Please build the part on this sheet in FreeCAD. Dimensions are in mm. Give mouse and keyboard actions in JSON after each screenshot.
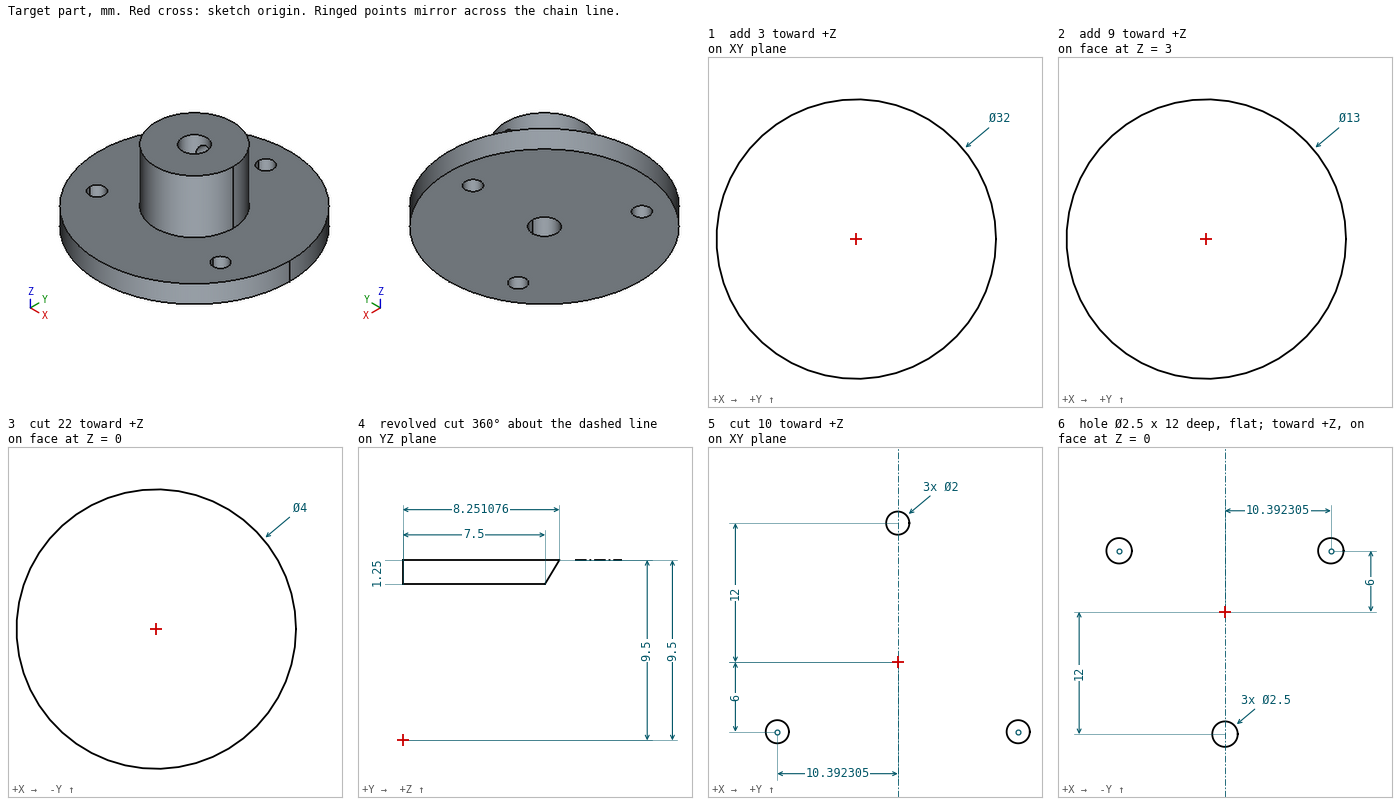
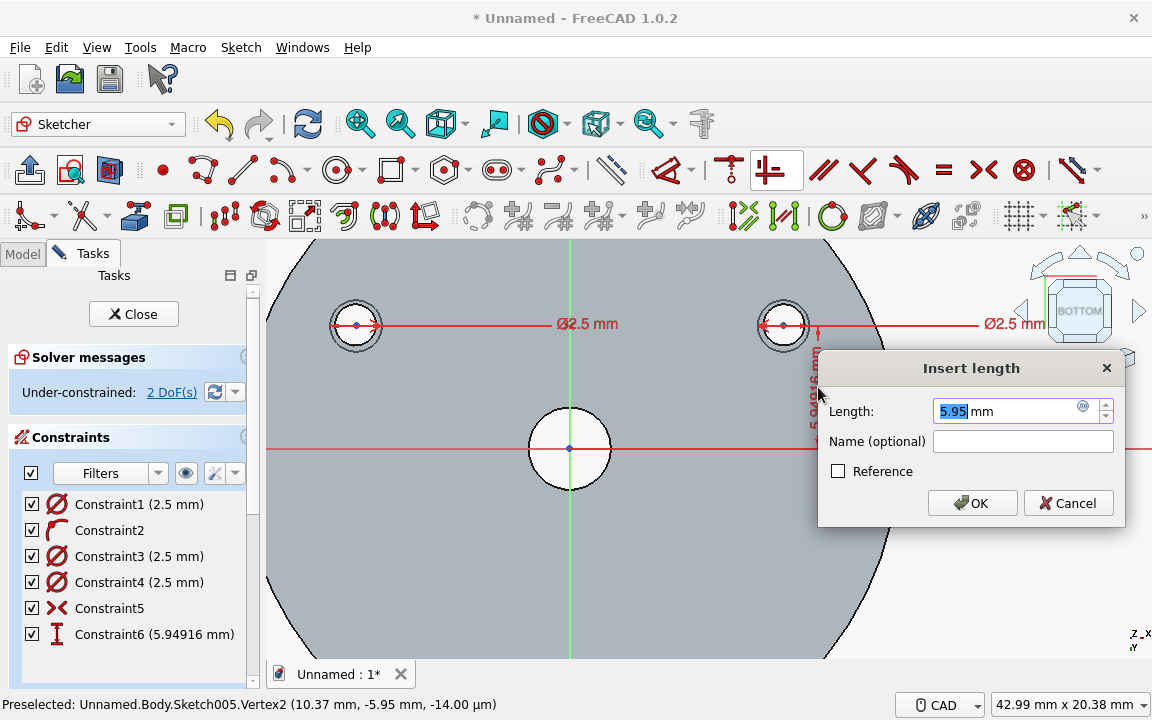
{"action": "type", "text": "6"}
{"action": "key", "text": "Return"}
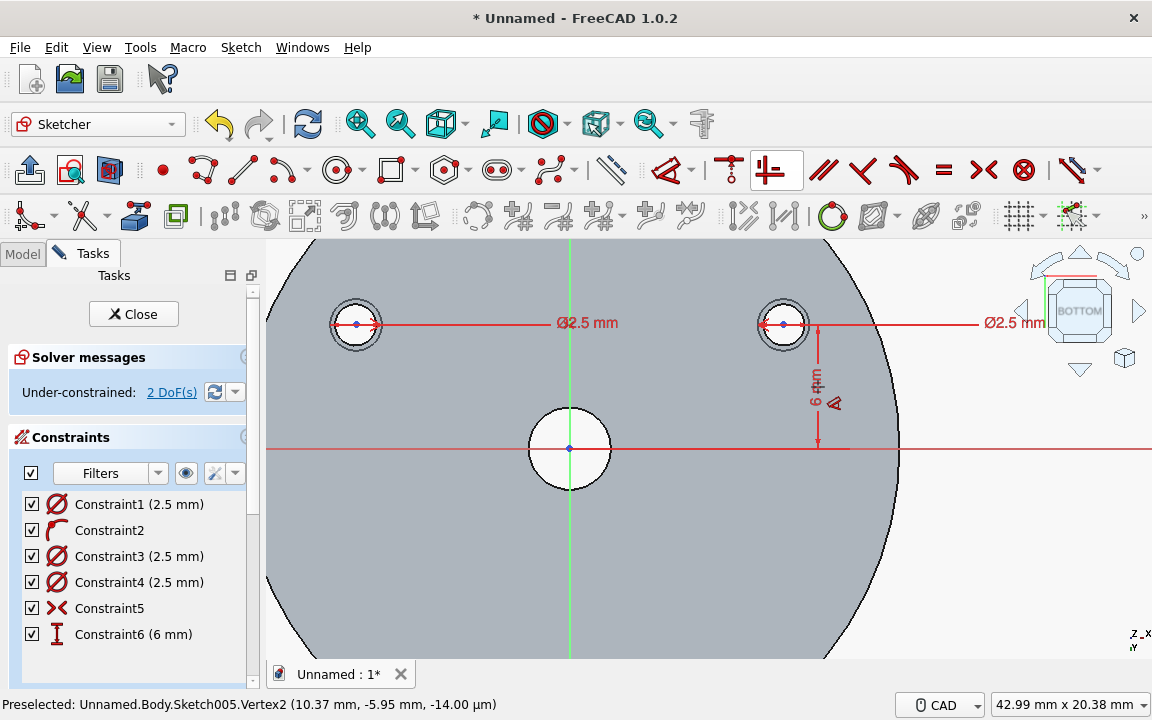
{"action": "scroll", "coordinate": [784, 324], "scroll_direction": "down", "scroll_amount": 2}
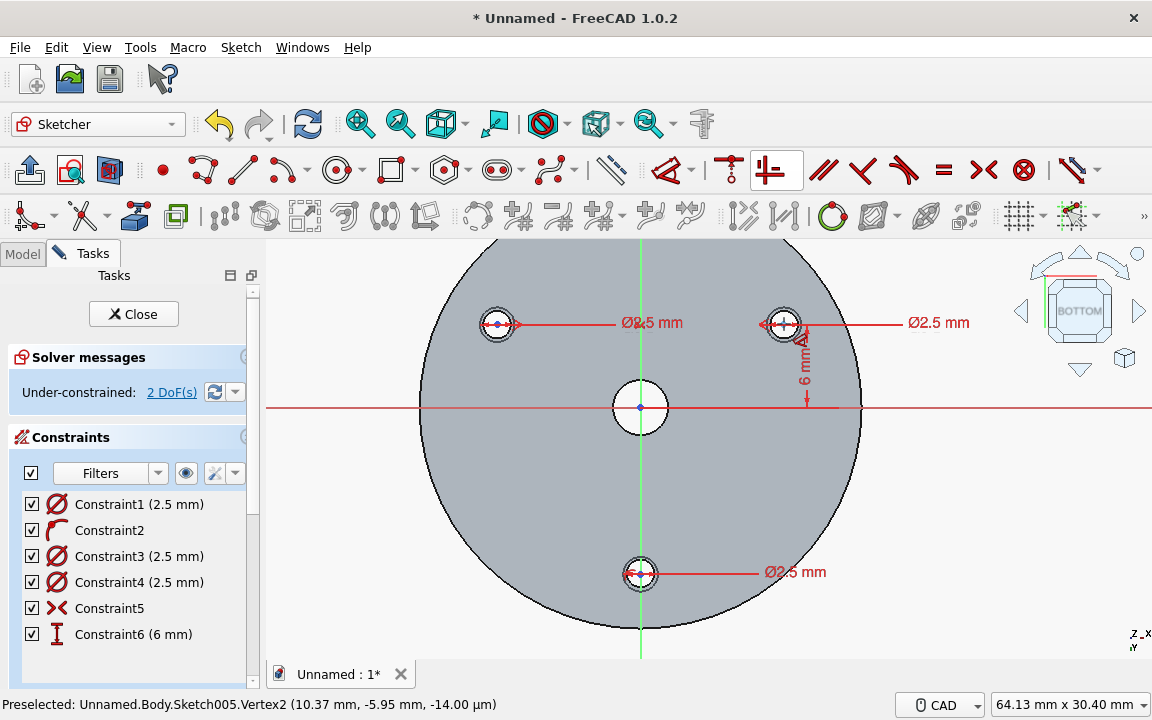
{"action": "left_click", "coordinate": [641, 574]}
{"action": "left_click", "coordinate": [675, 491]}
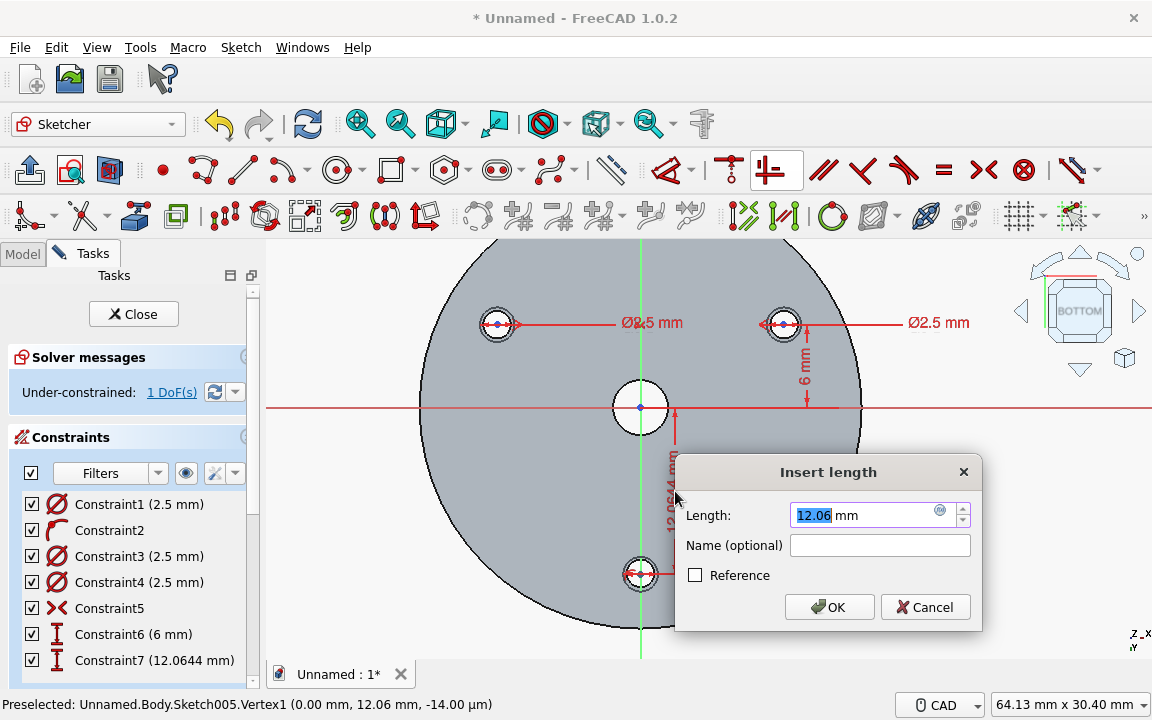
{"action": "type", "text": "12"}
{"action": "key", "text": "Return"}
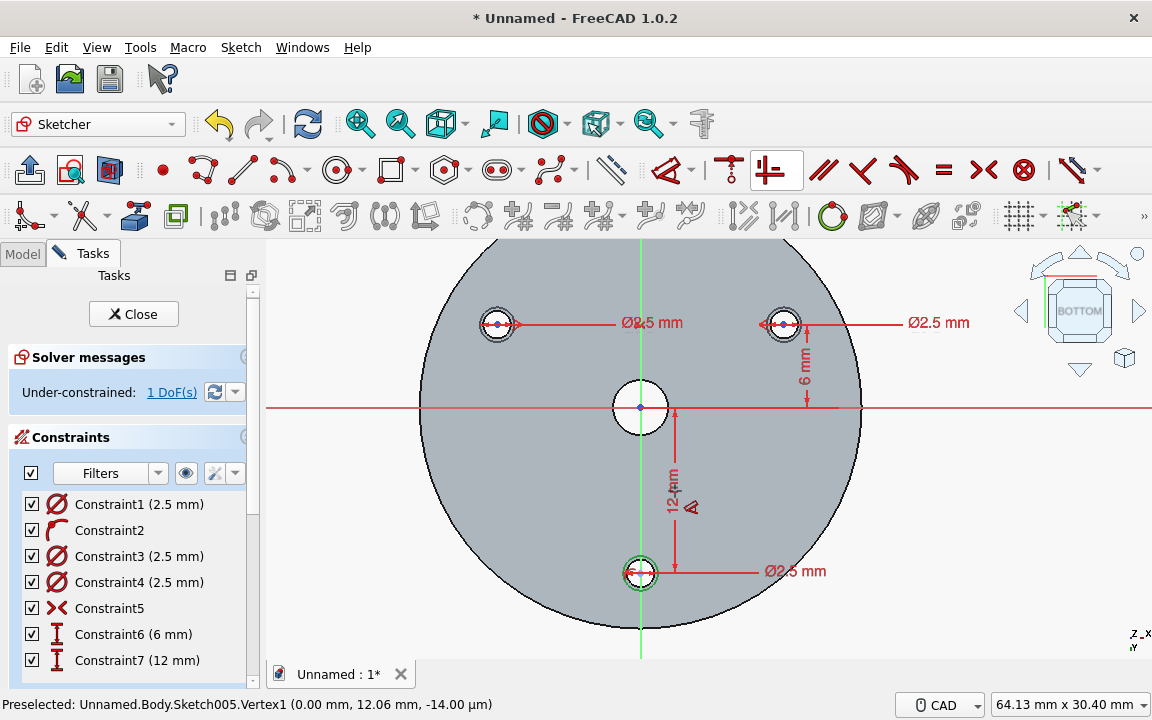
{"action": "left_click", "coordinate": [784, 325]}
{"action": "left_click", "coordinate": [712, 291]}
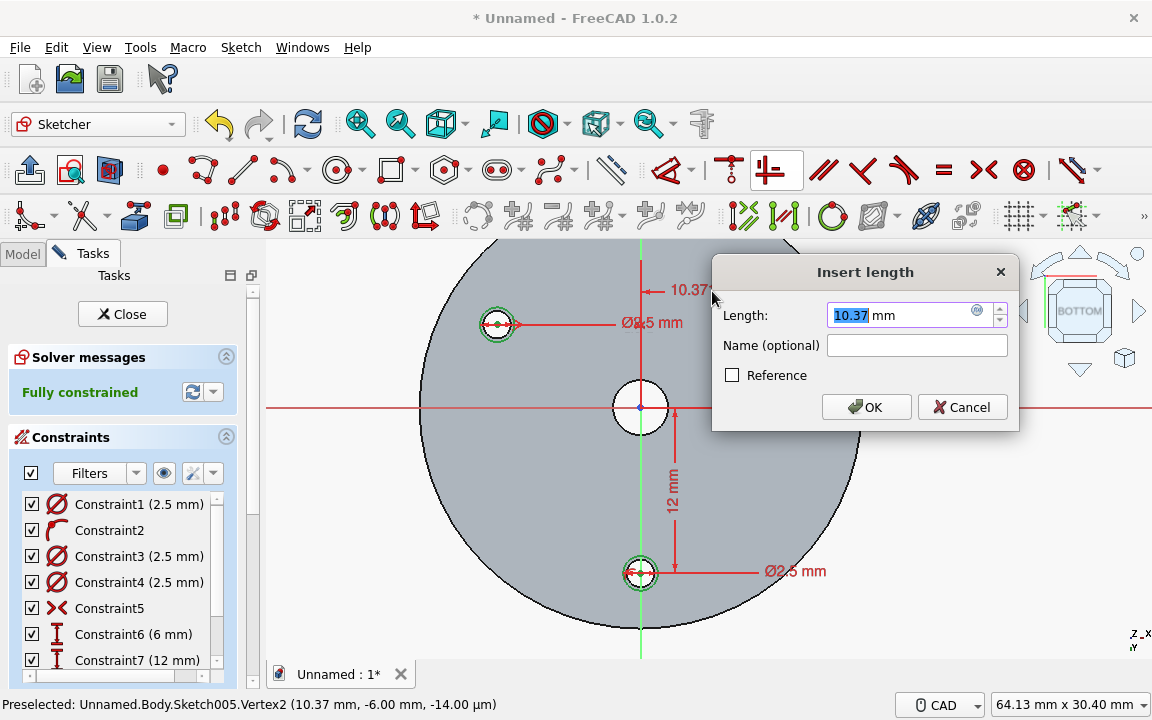
{"action": "type", "text": "10.392305"}
{"action": "key", "text": "Return"}
{"action": "key", "text": "Escape"}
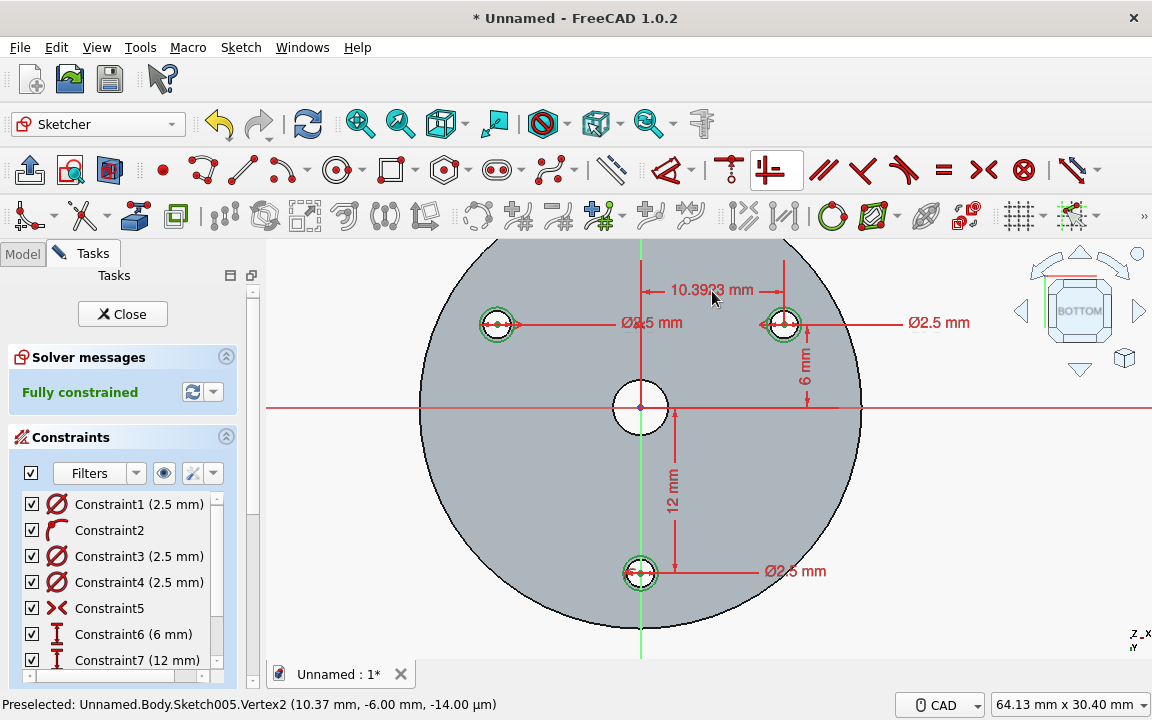
{"action": "left_click", "coordinate": [123, 314]}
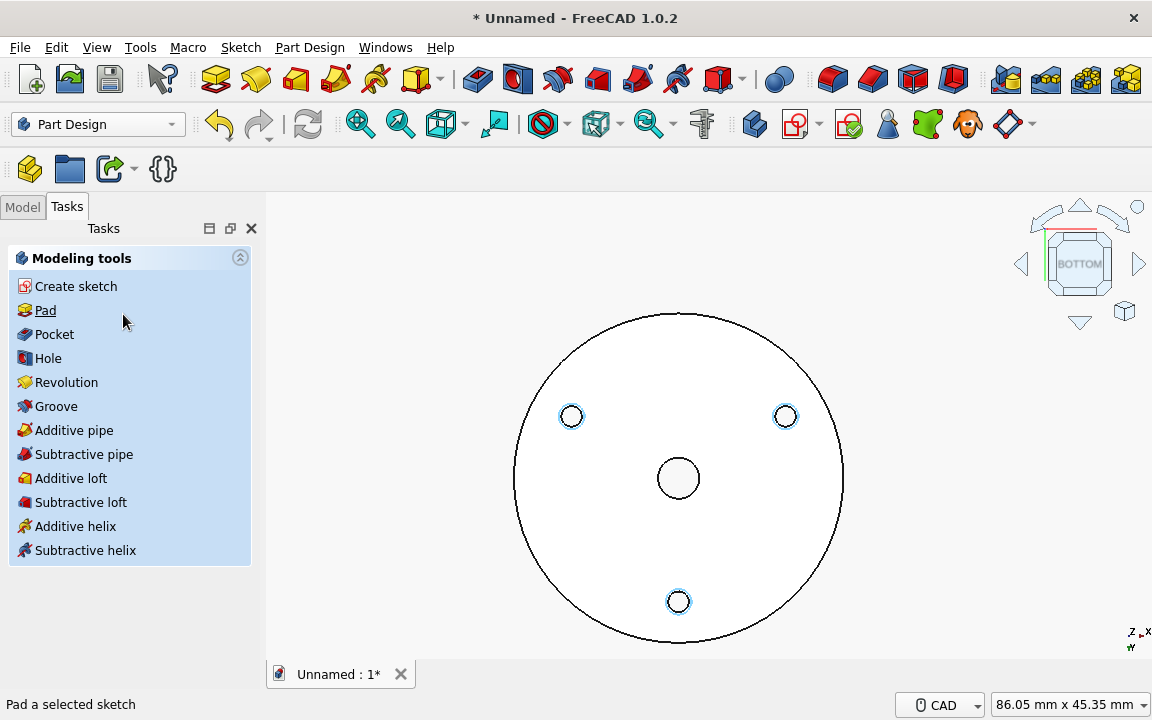
{"action": "left_click", "coordinate": [518, 80]}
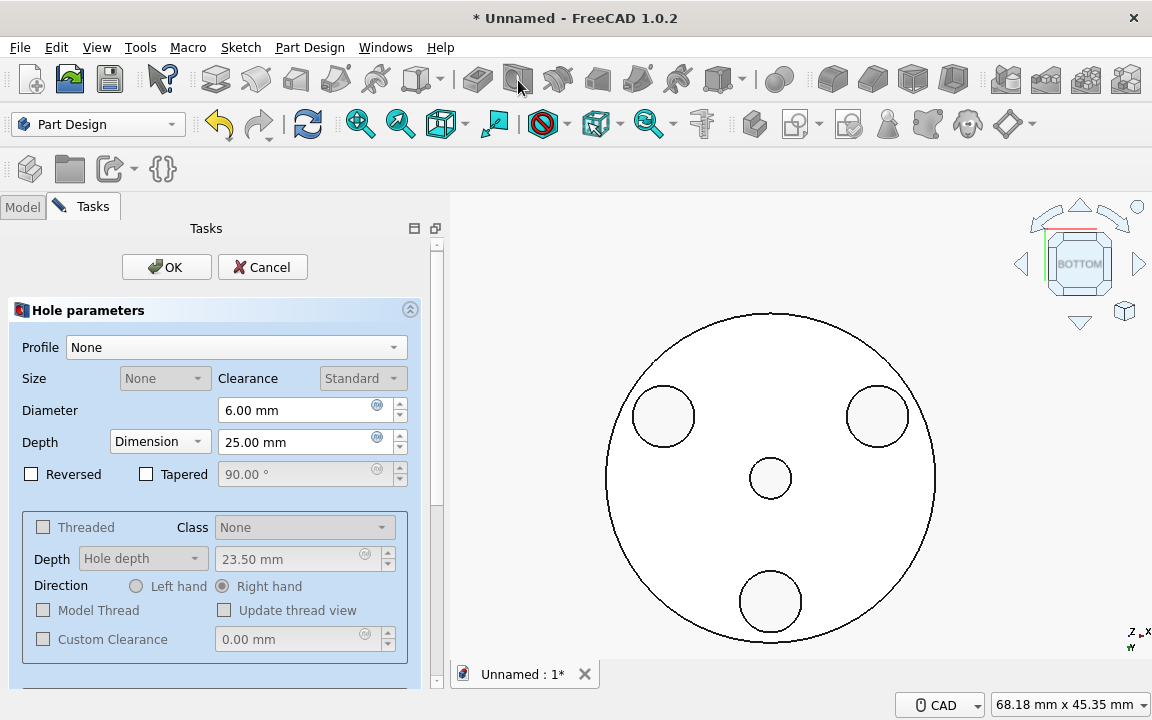
{"action": "triple_click", "coordinate": [305, 410]}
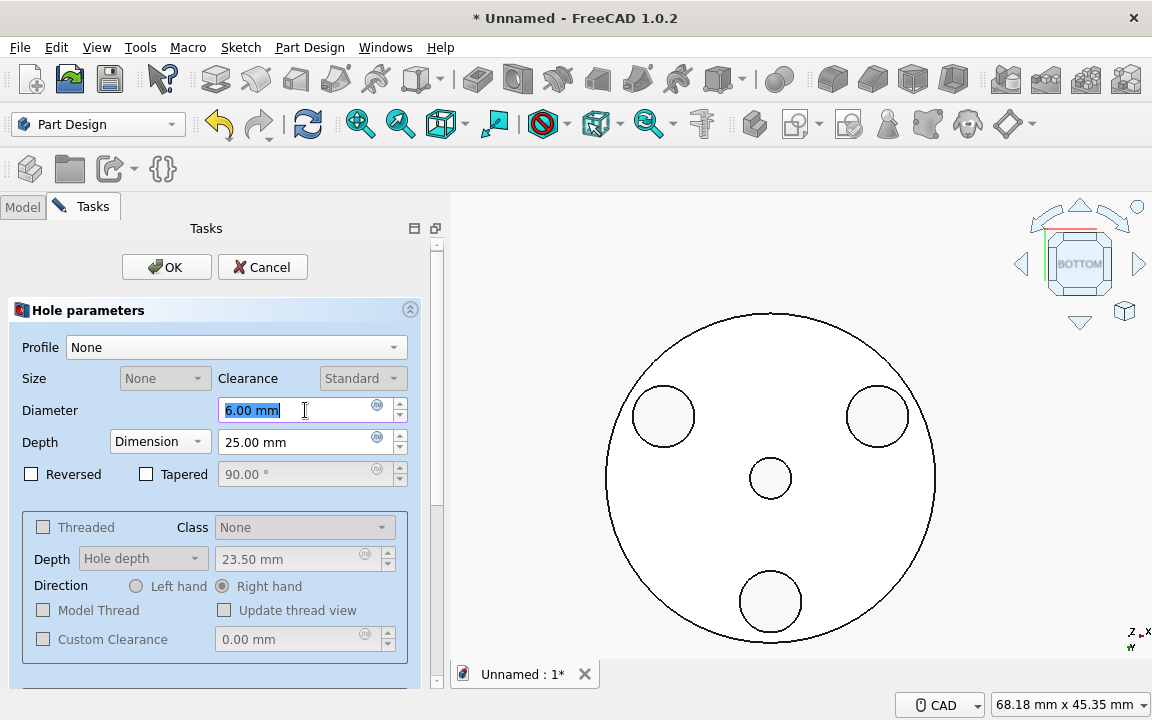
{"action": "type", "text": "2.5"}
{"action": "key", "text": "Tab"}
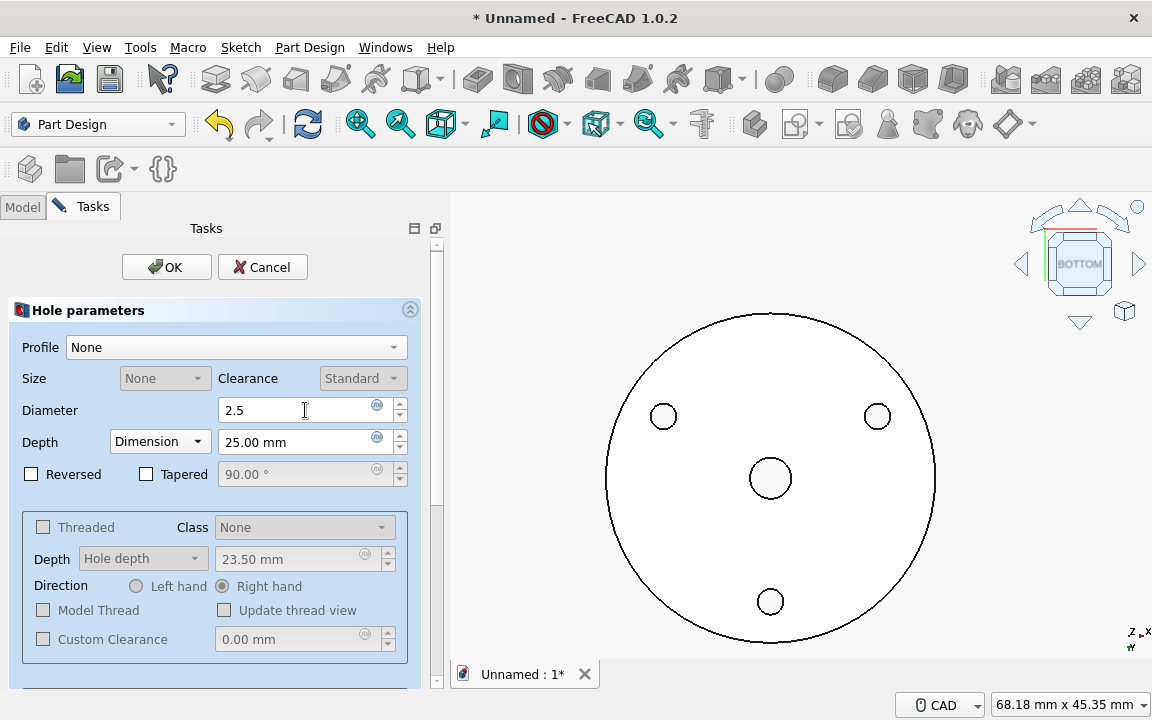
{"action": "triple_click", "coordinate": [305, 442]}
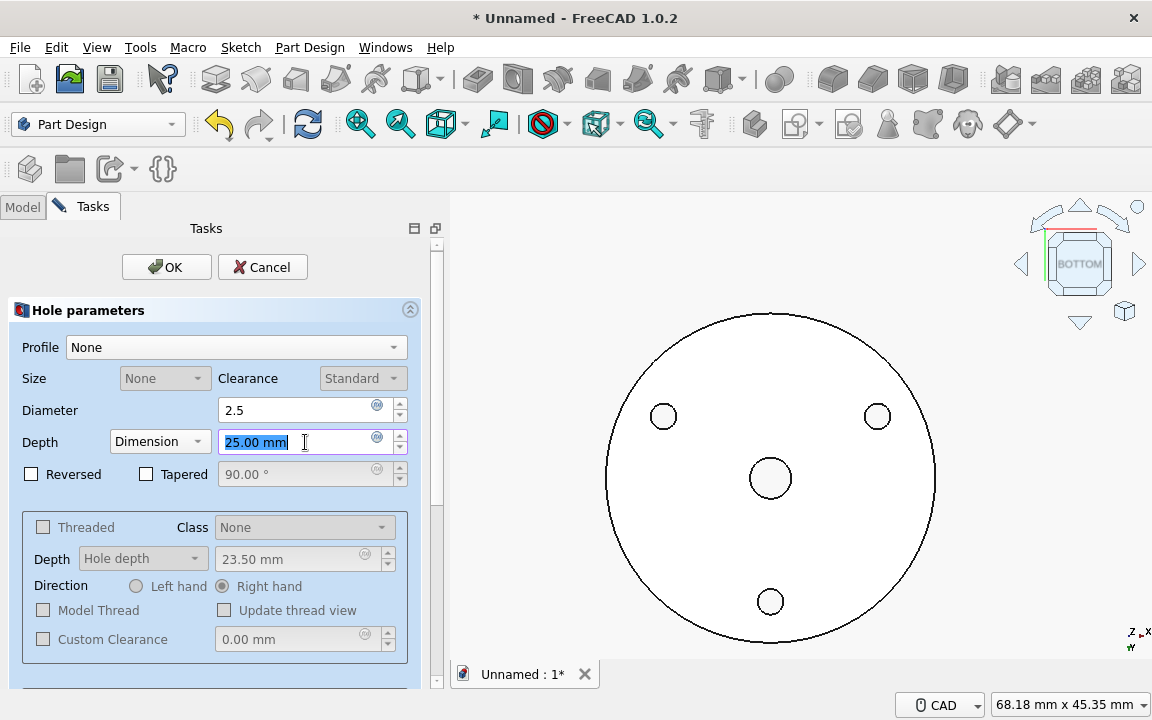
{"action": "type", "text": "12"}
{"action": "key", "text": "Tab"}